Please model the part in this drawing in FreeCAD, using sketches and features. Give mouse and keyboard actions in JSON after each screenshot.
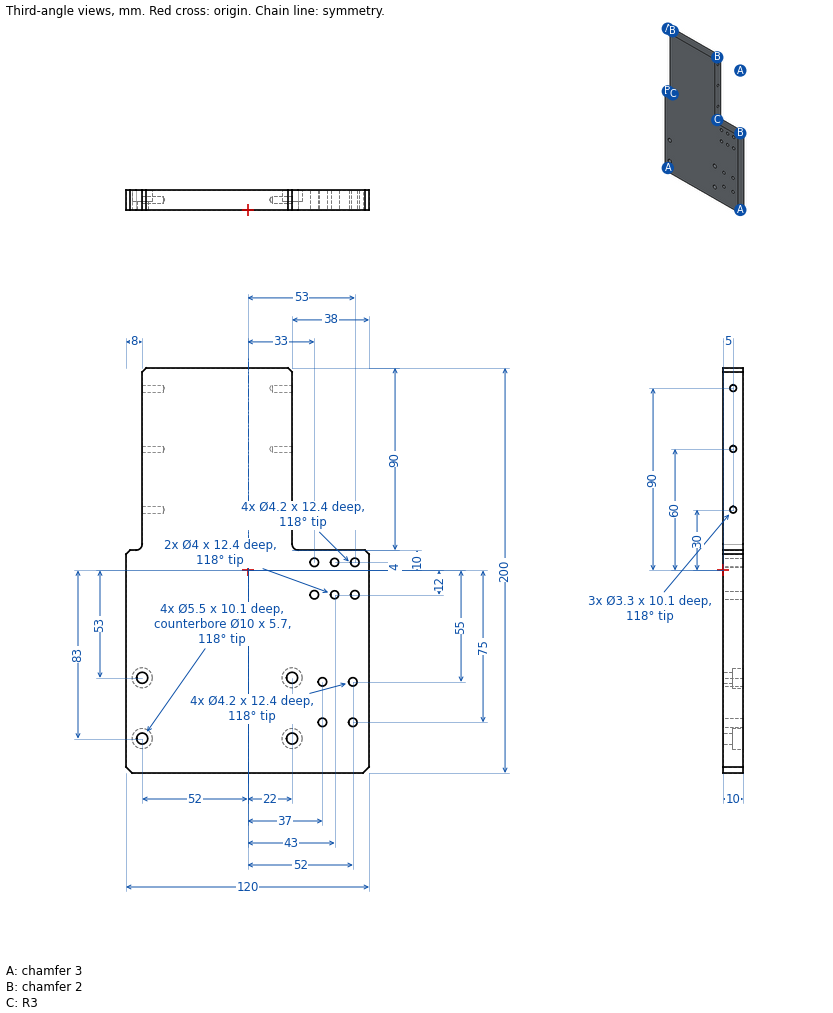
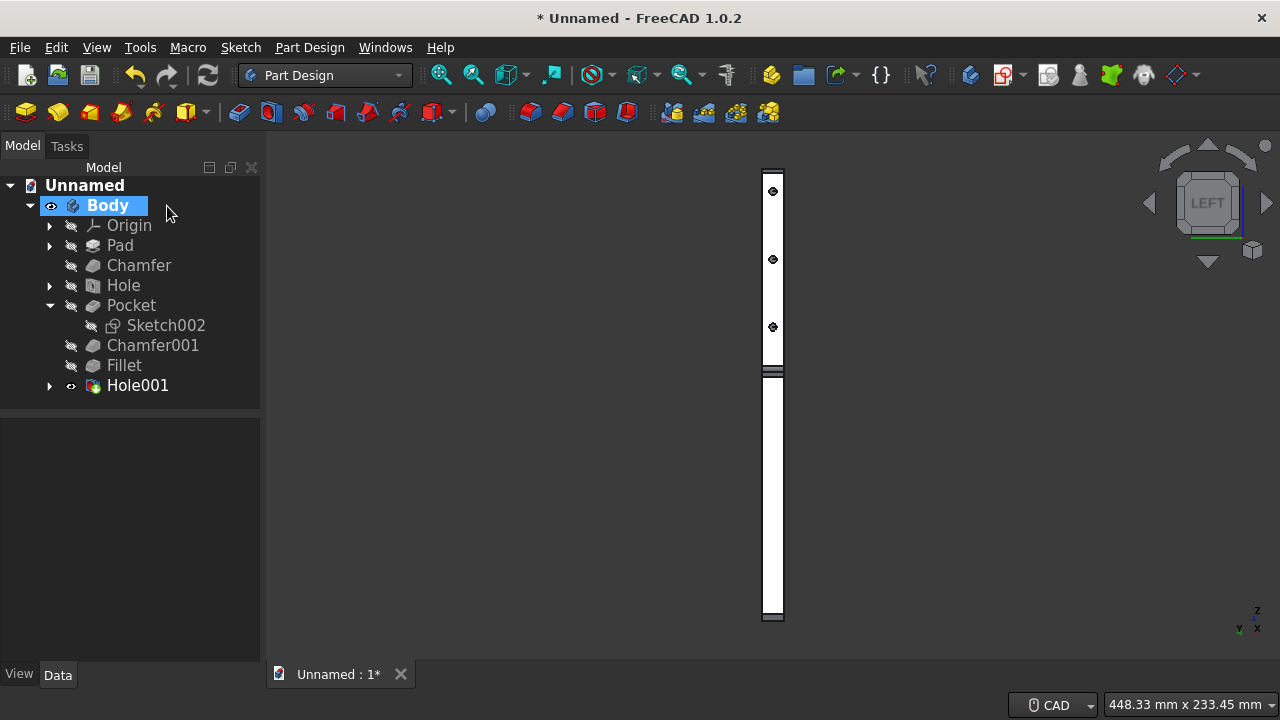
{"action": "key", "text": "0"}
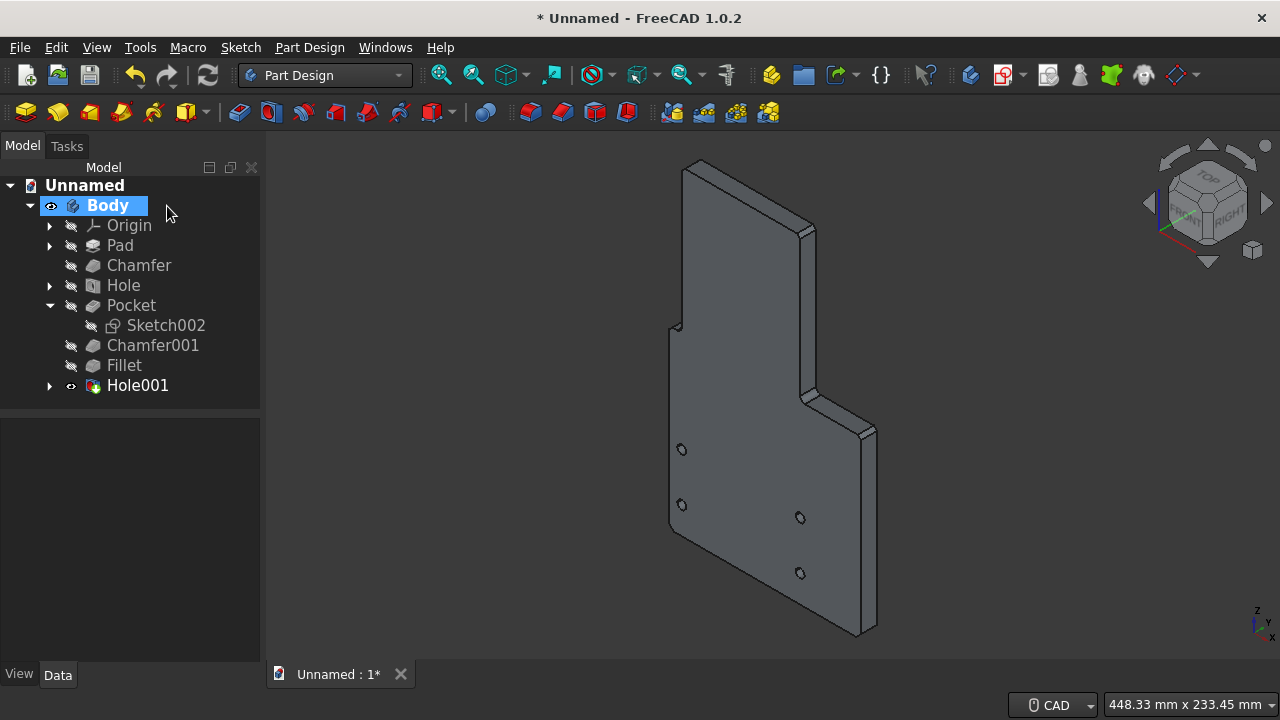
{"action": "key", "text": "3"}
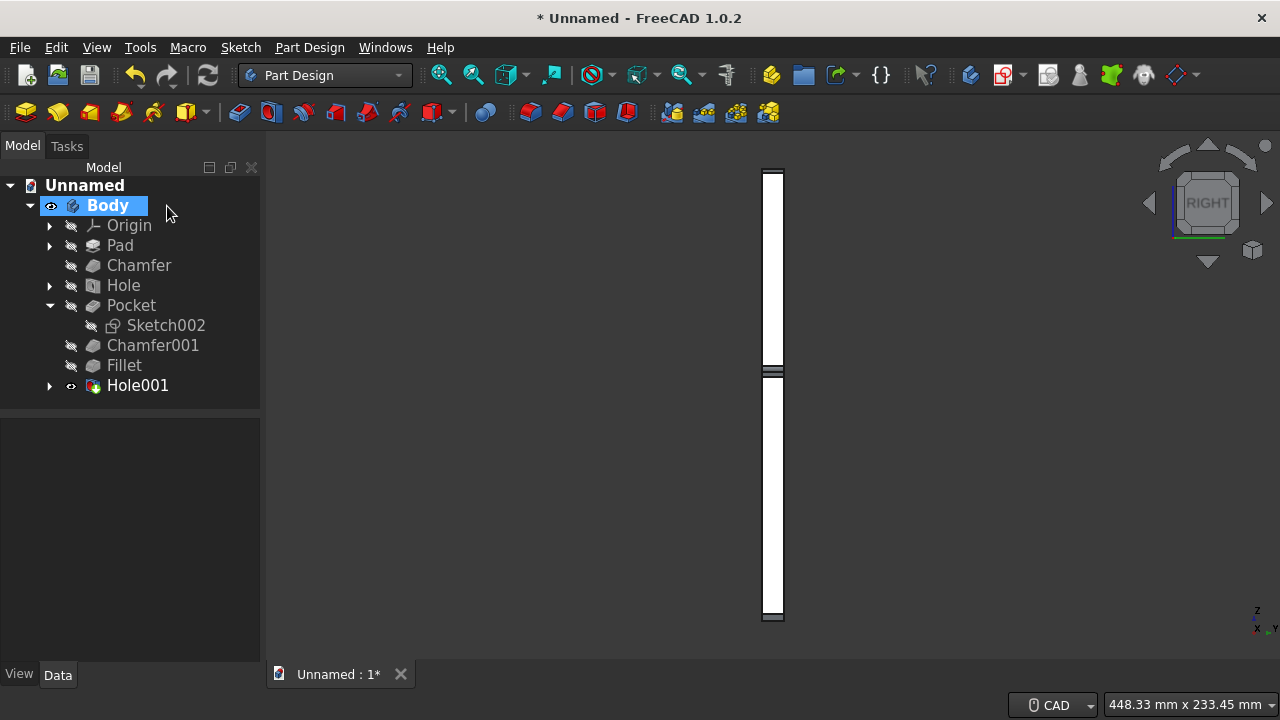
{"action": "left_click", "coordinate": [773, 241]}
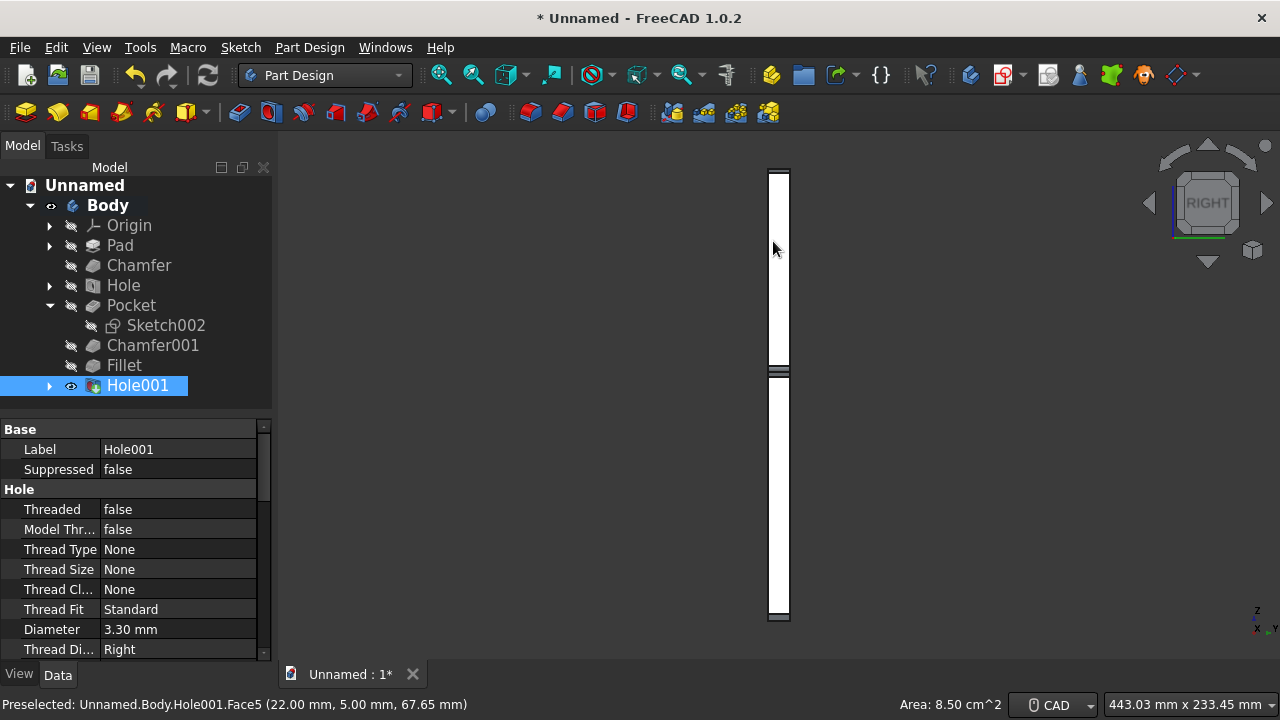
{"action": "left_click", "coordinate": [1004, 76]}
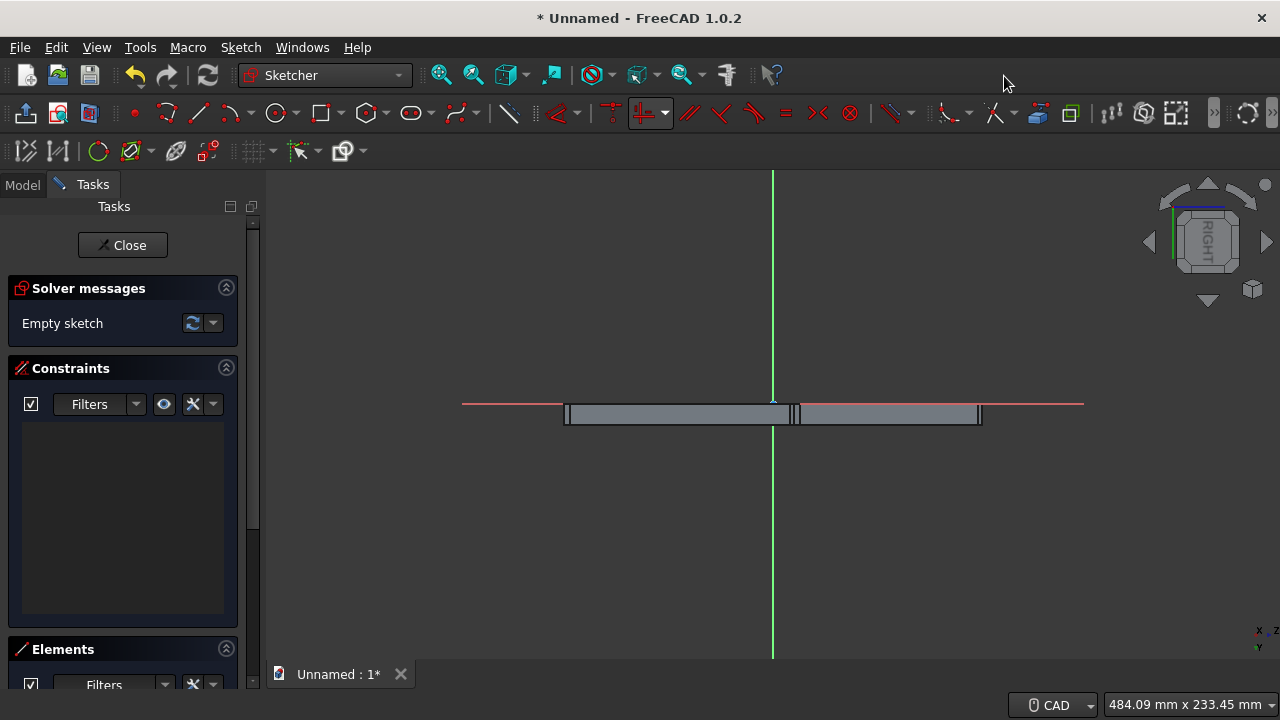
{"action": "scroll", "coordinate": [940, 409], "scroll_direction": "up", "scroll_amount": 6}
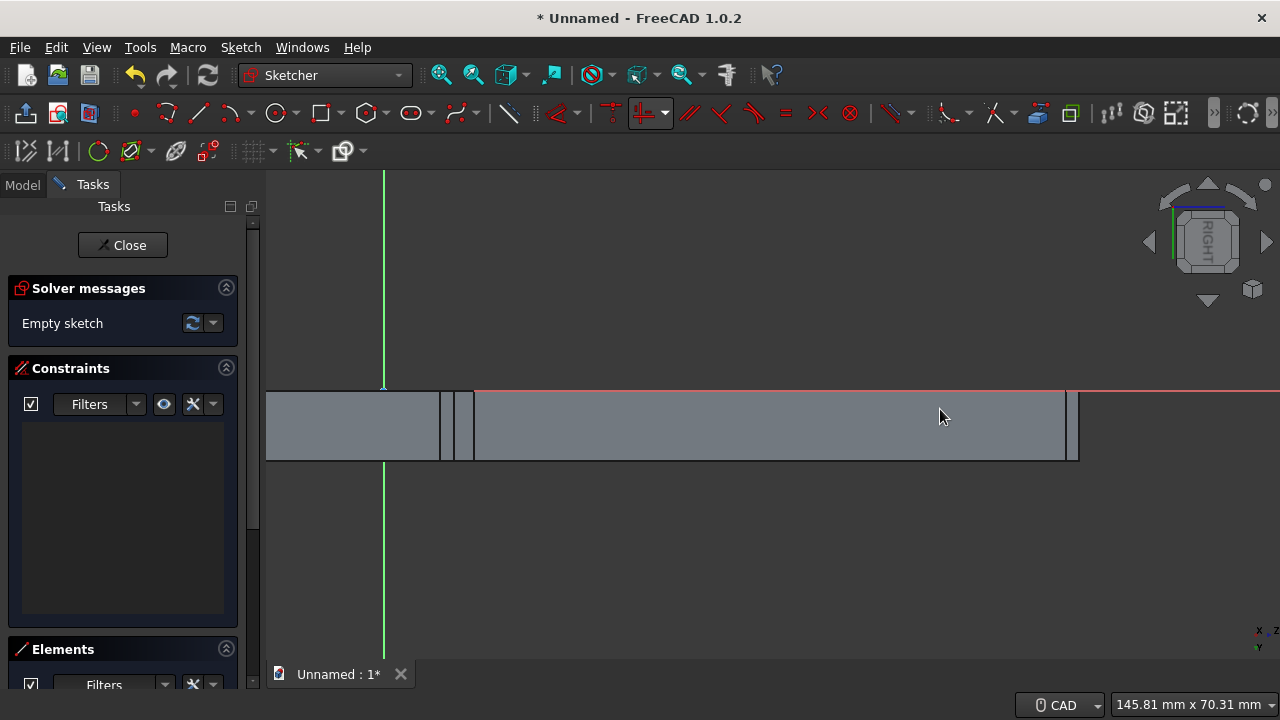
{"action": "left_click", "coordinate": [276, 114]}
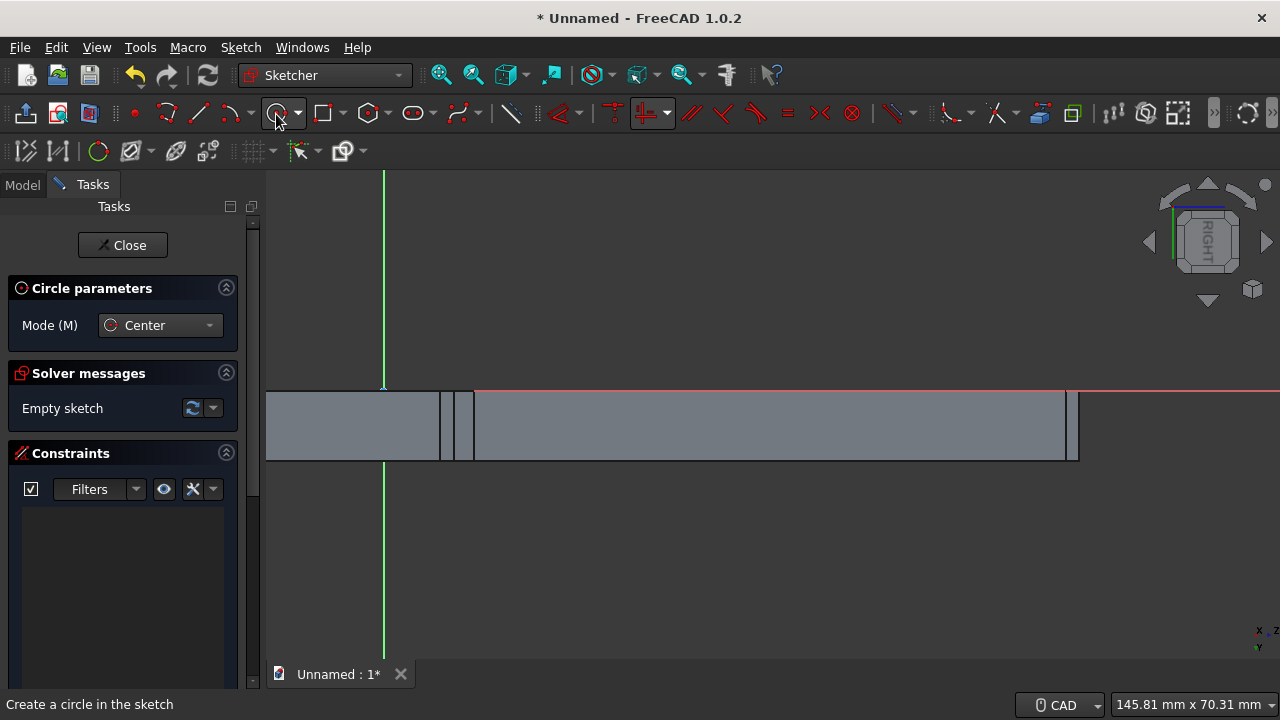
{"action": "scroll", "coordinate": [593, 426], "scroll_direction": "up", "scroll_amount": 4}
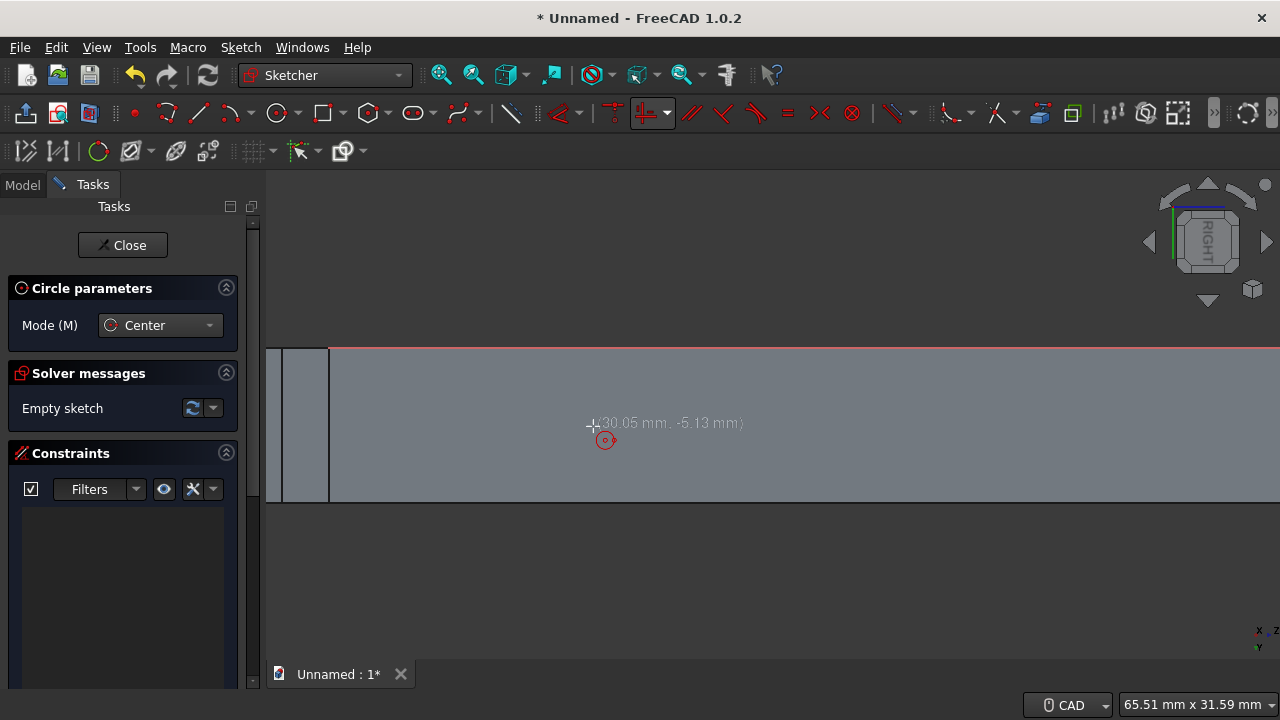
{"action": "left_click", "coordinate": [592, 426]}
{"action": "left_click", "coordinate": [610, 408]}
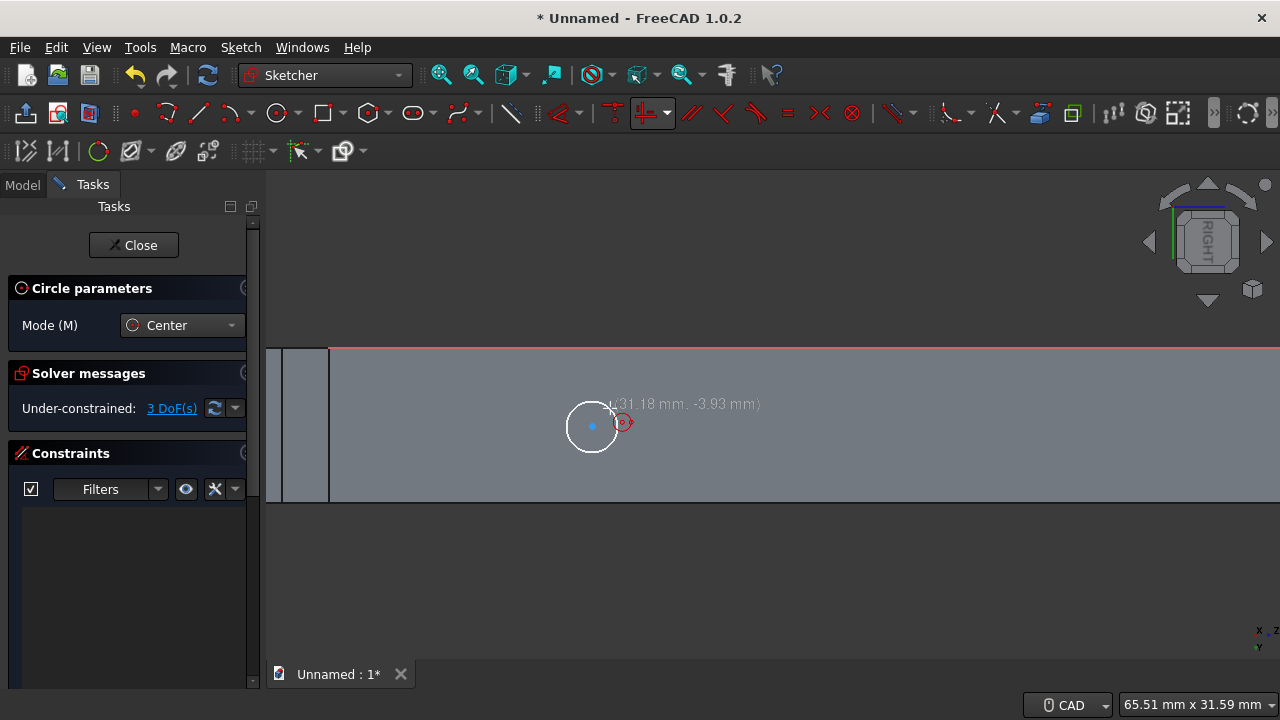
{"action": "left_click", "coordinate": [1056, 426]}
{"action": "left_click", "coordinate": [1074, 408]}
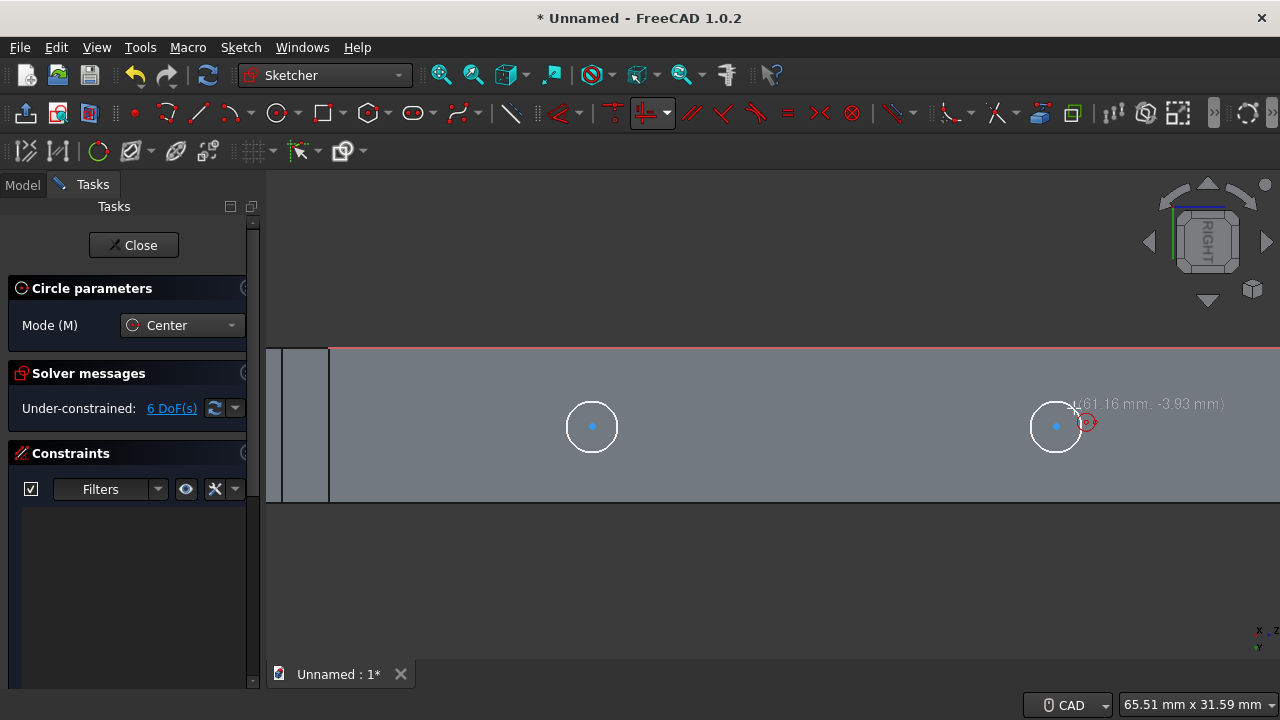
{"action": "scroll", "coordinate": [597, 427], "scroll_direction": "down", "scroll_amount": 4}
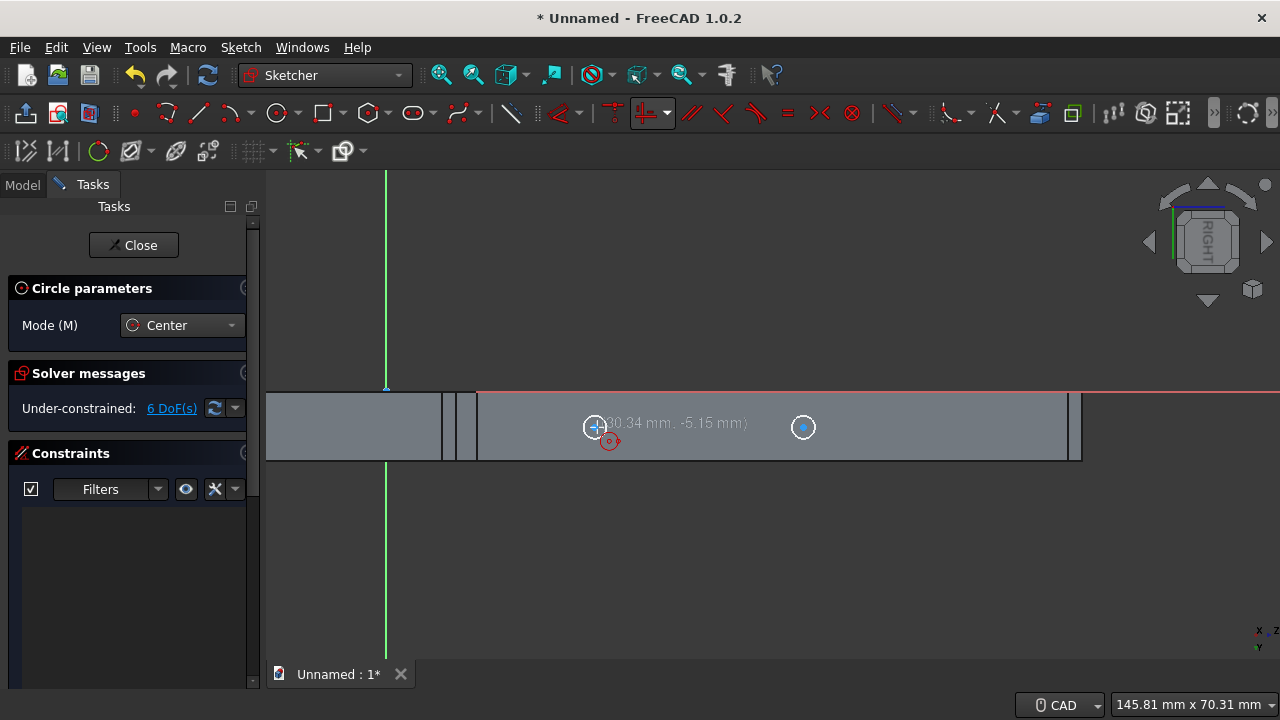
{"action": "scroll", "coordinate": [1012, 427], "scroll_direction": "up", "scroll_amount": 4}